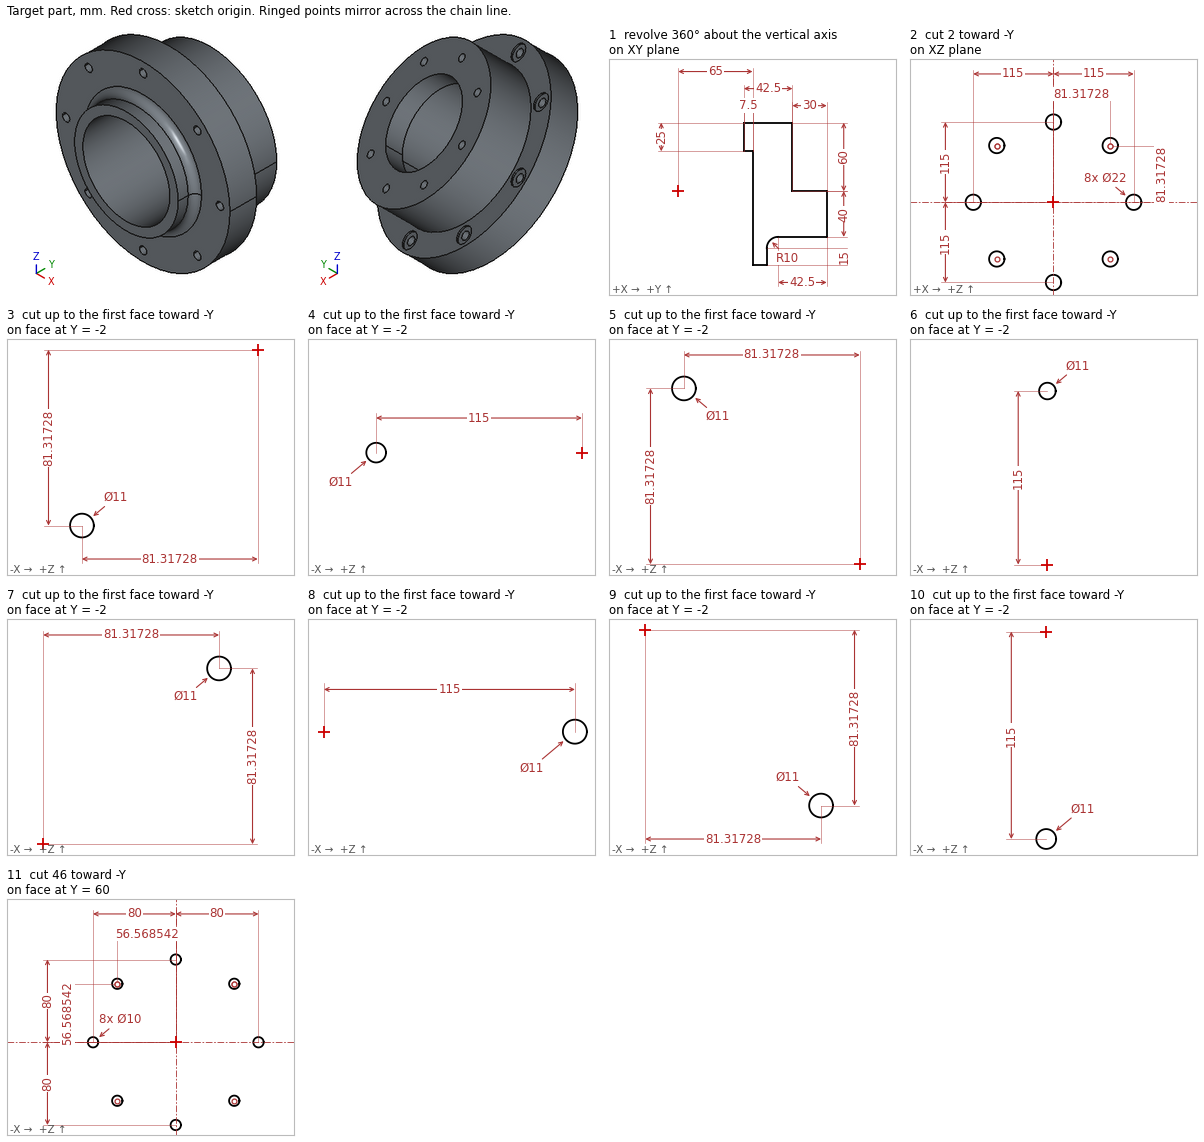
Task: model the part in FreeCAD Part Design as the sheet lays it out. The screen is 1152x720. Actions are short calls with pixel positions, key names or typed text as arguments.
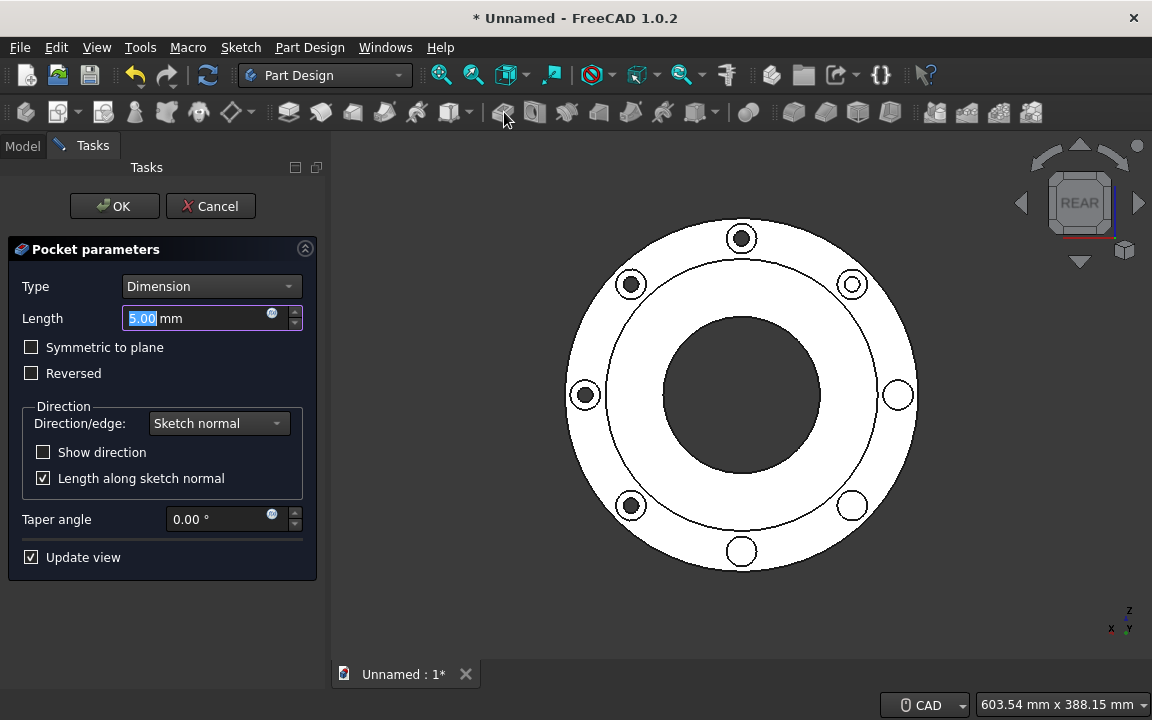
click(212, 286)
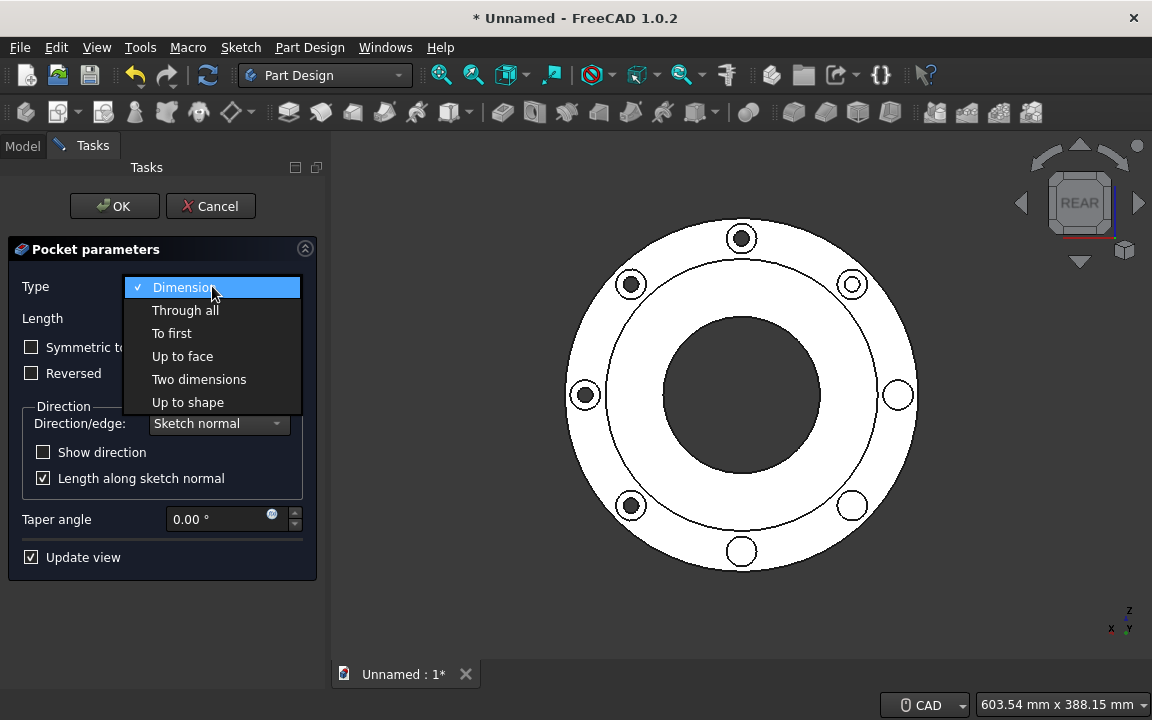
click(212, 334)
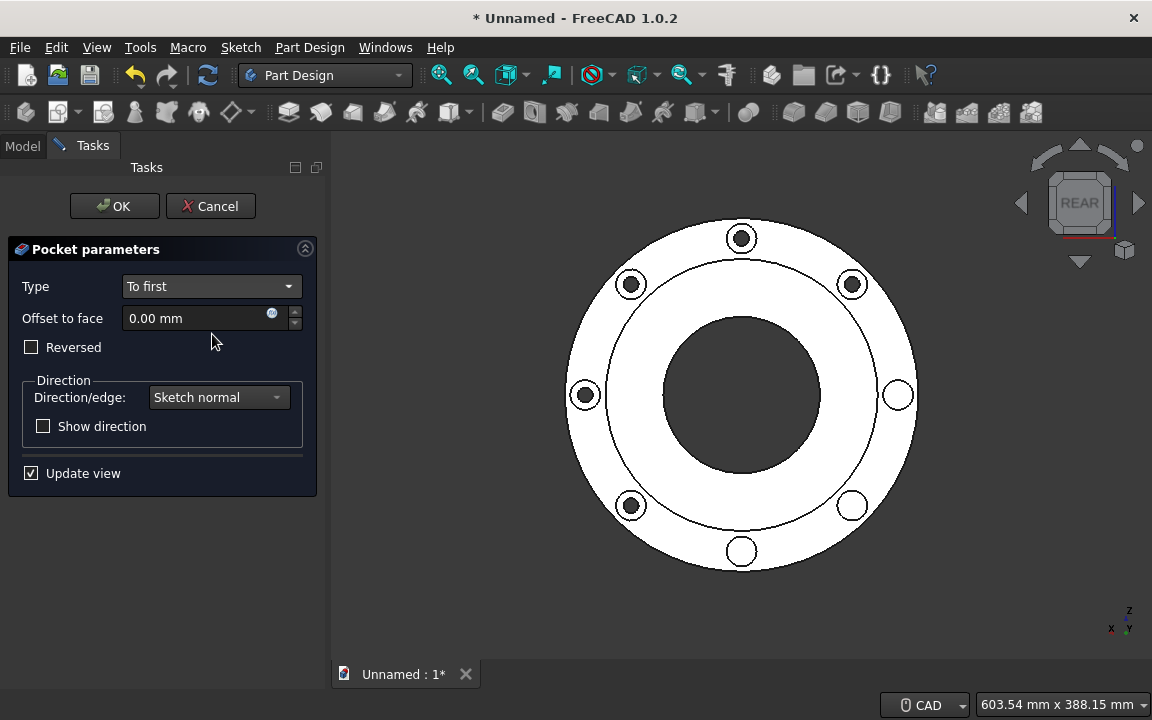
click(115, 206)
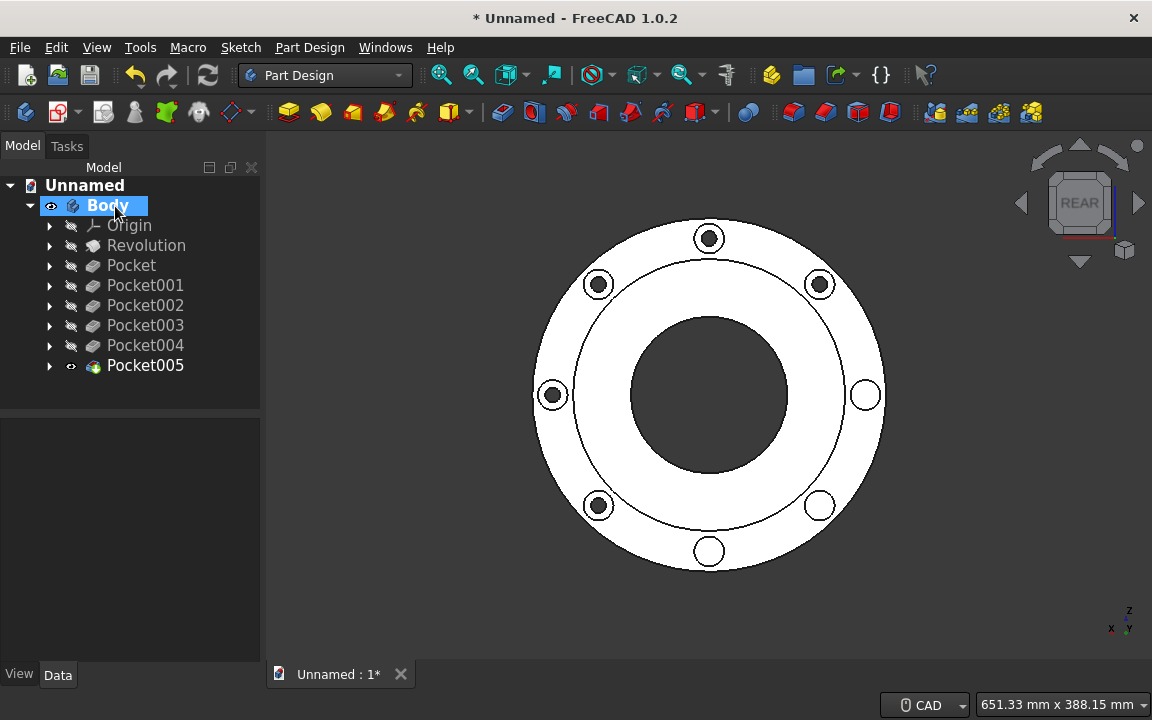
click(866, 394)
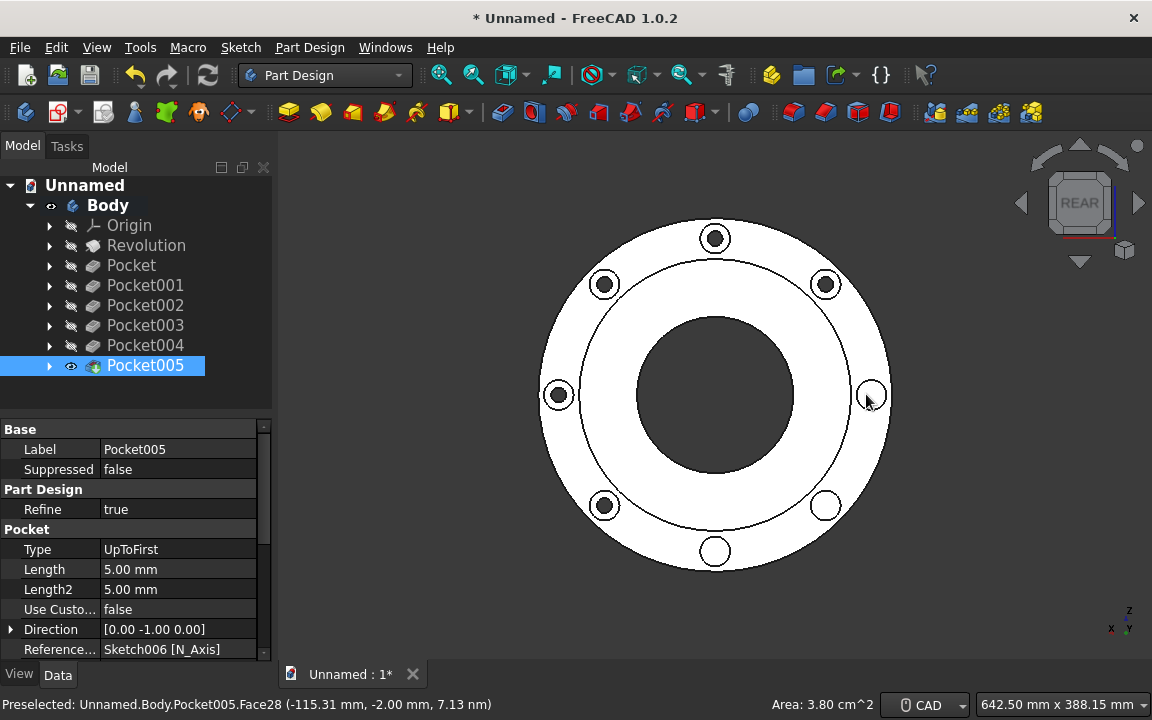
click(58, 112)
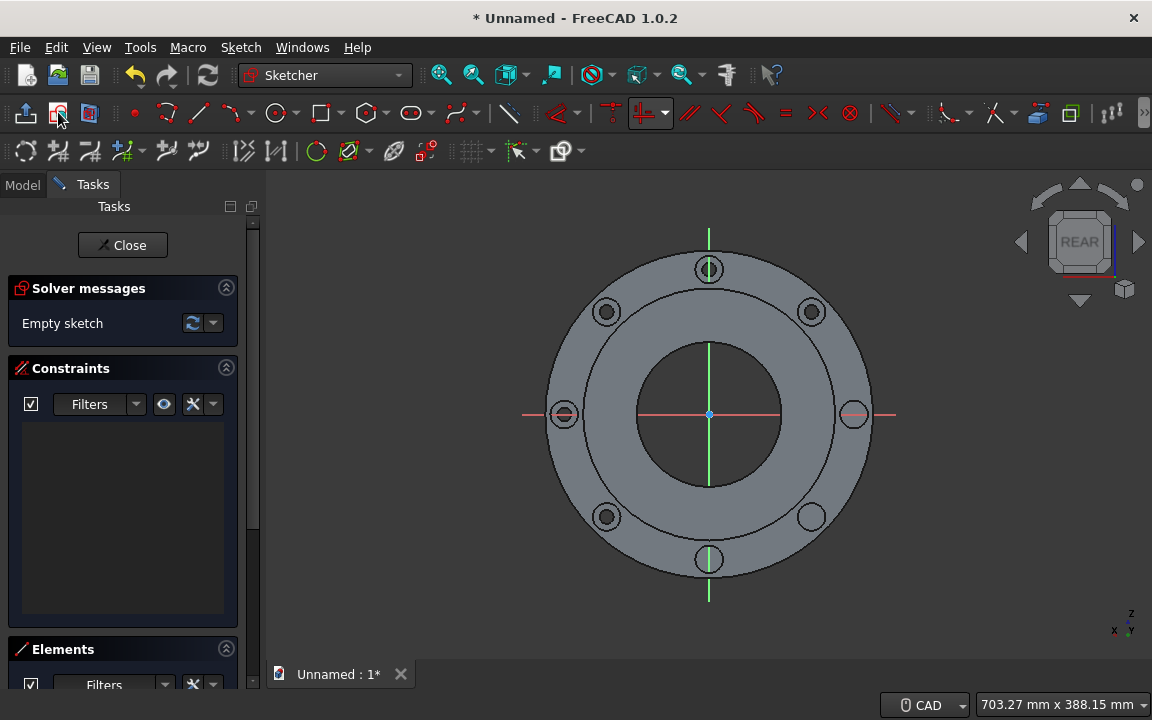
scroll(865, 415, up, 15)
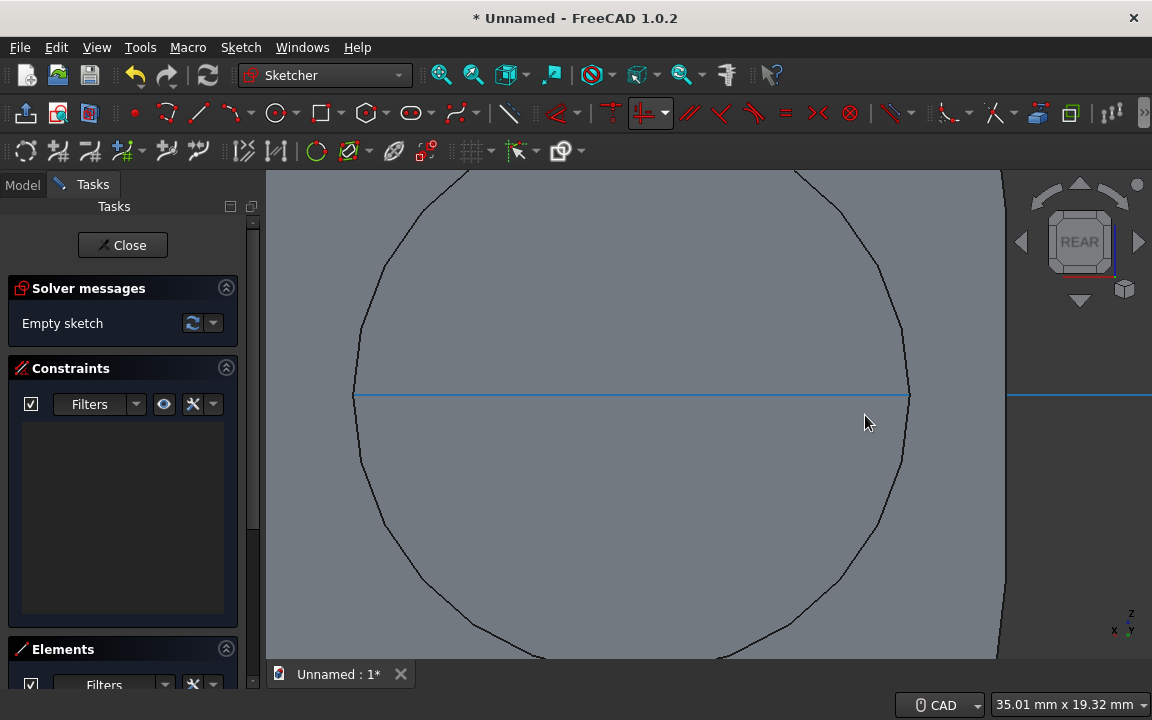
key(g)
key(c)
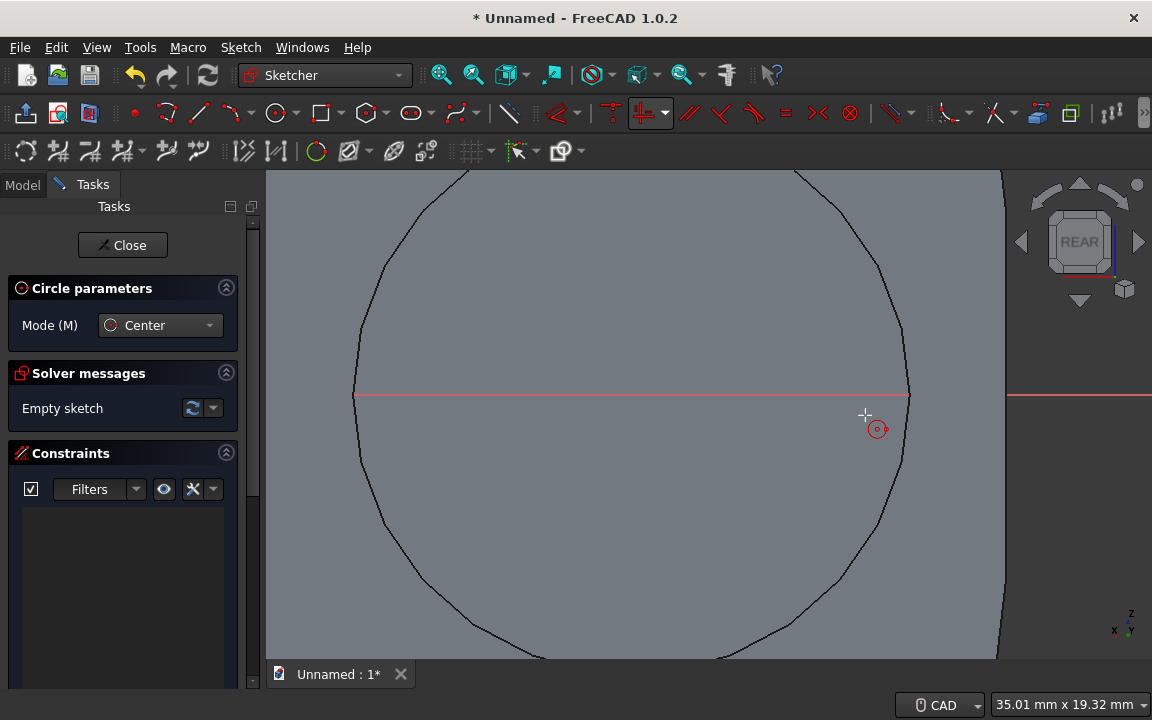
click(631, 395)
move(730, 297)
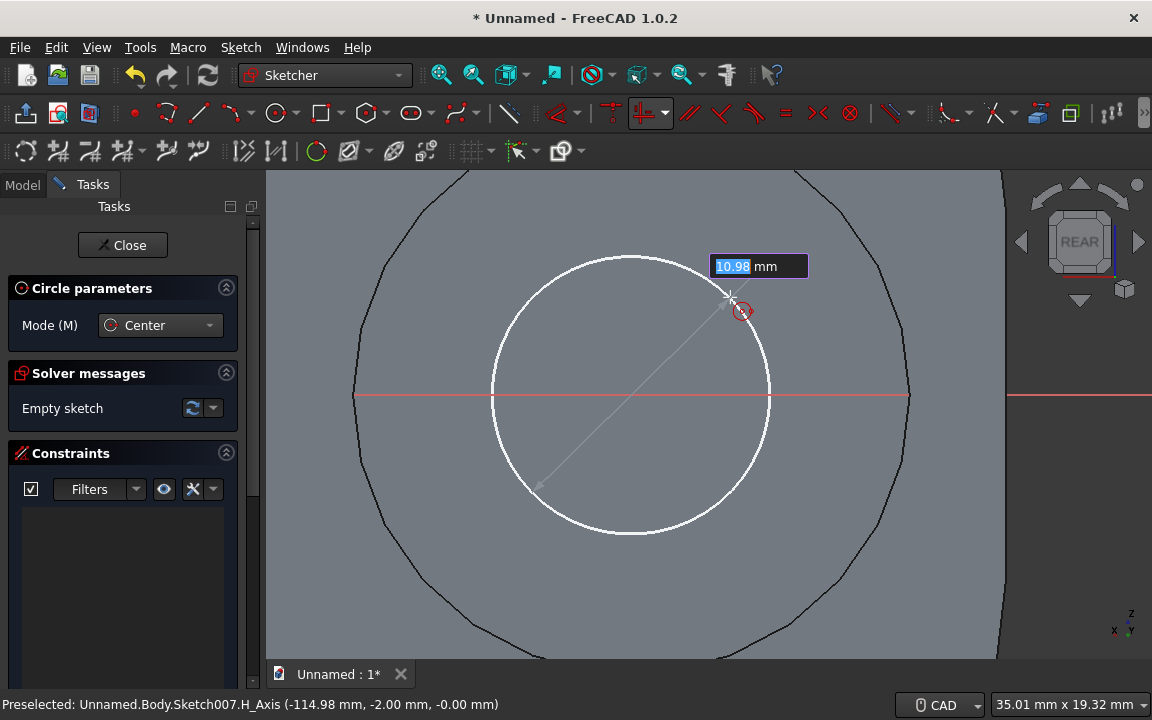
text(11)
key(Return)
key(Escape)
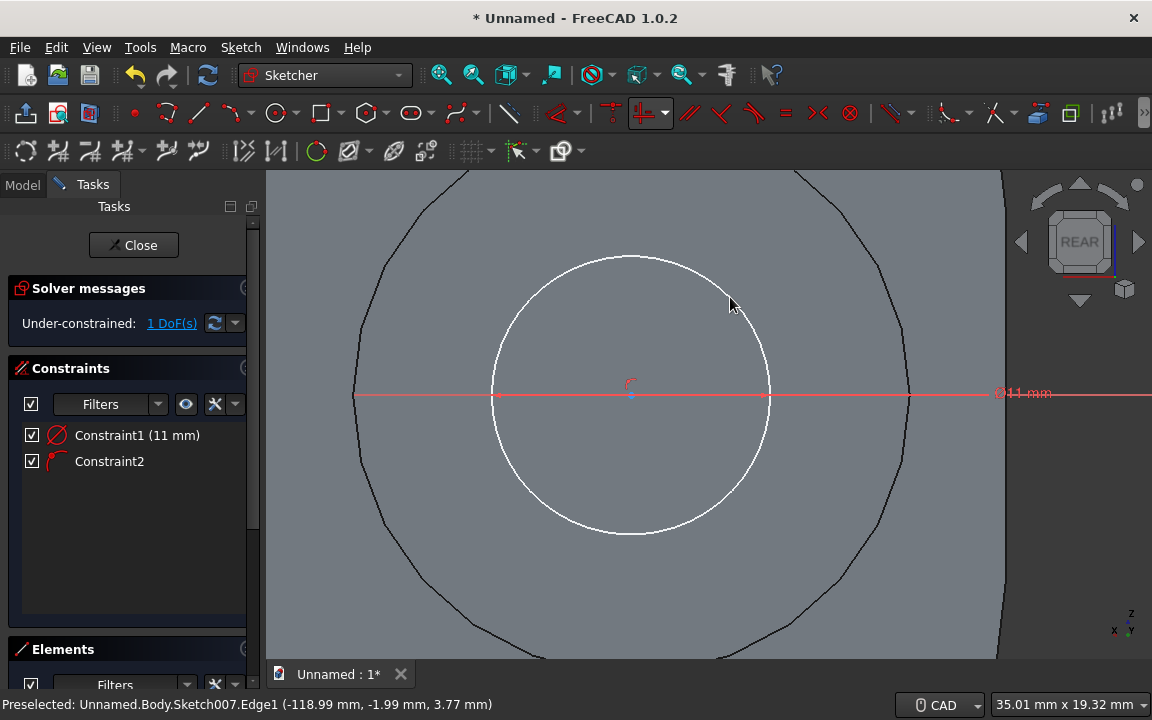
key(d)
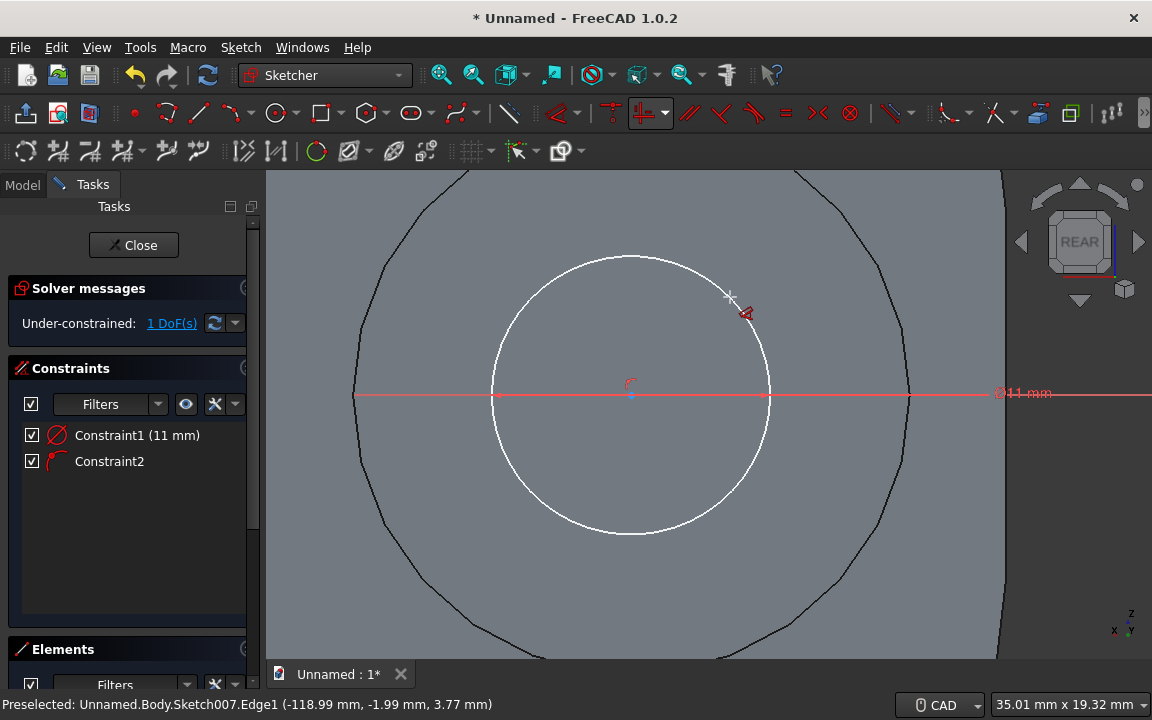
click(631, 395)
click(462, 429)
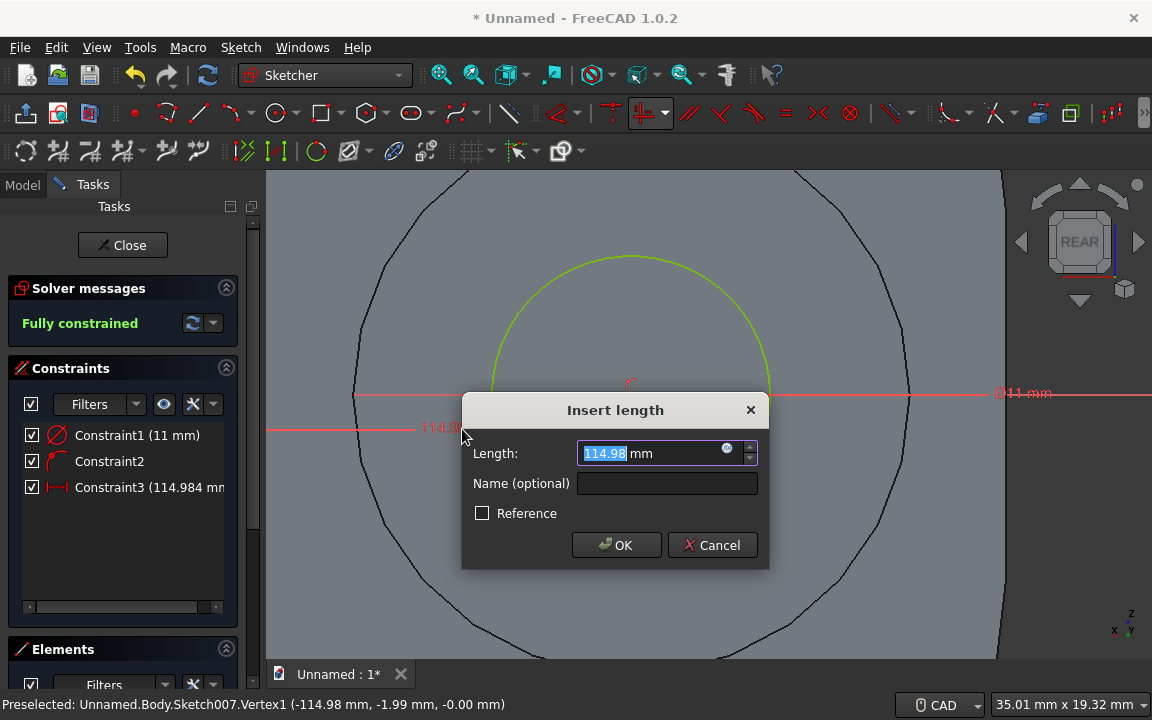
text(115)
key(Return)
key(Escape)